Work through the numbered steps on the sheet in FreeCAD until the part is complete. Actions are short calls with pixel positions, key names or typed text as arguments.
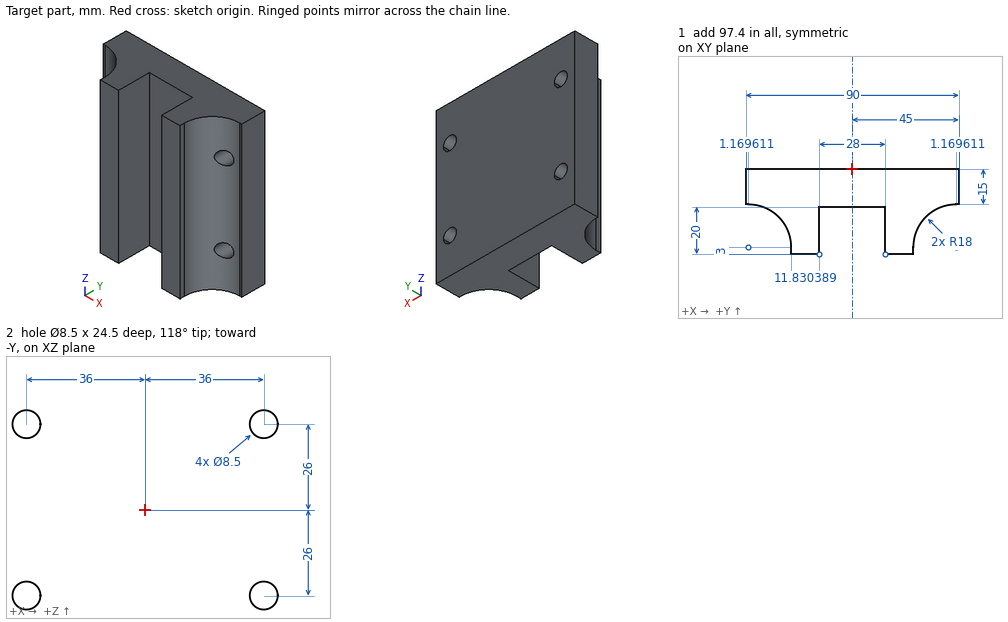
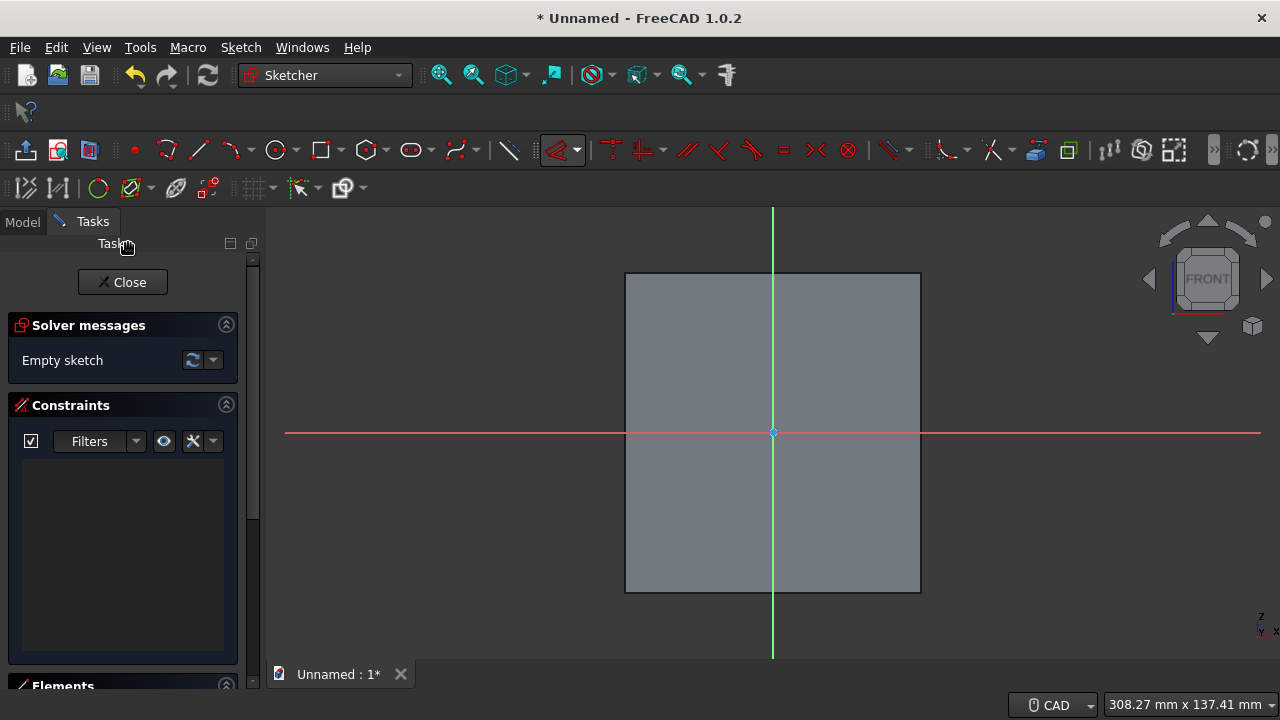
scroll(912, 433, up, 2)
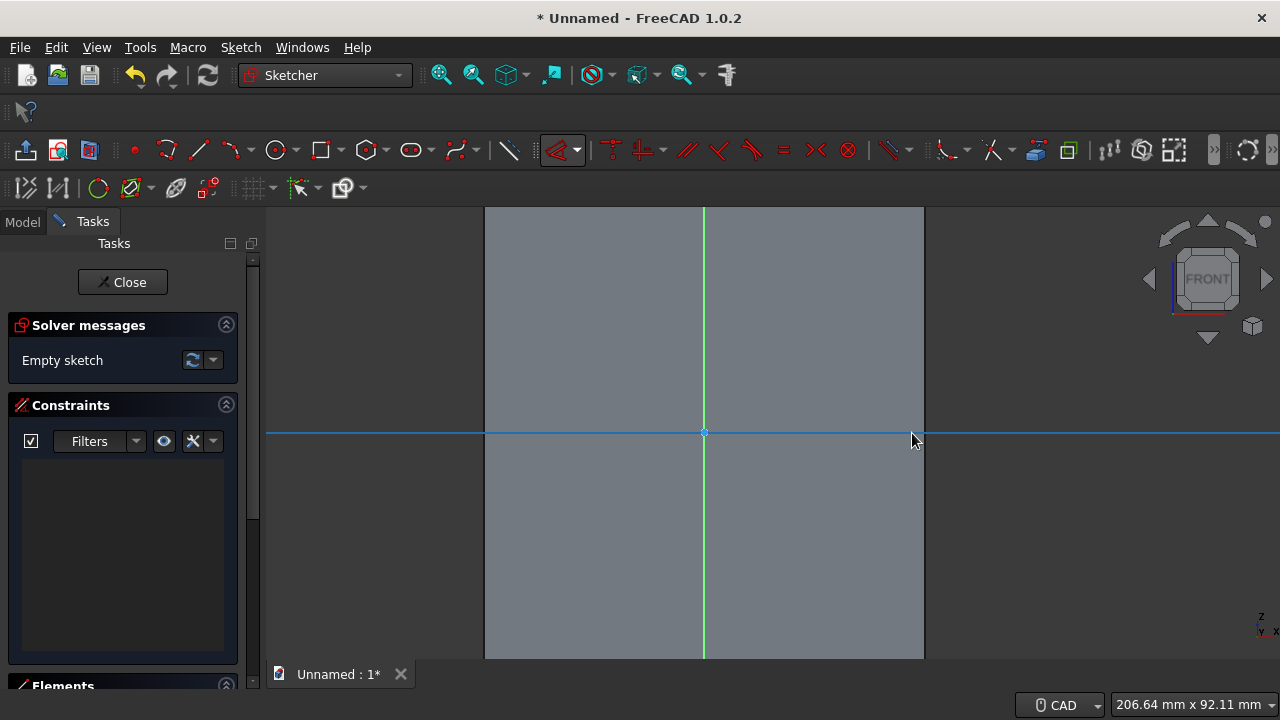
click(276, 150)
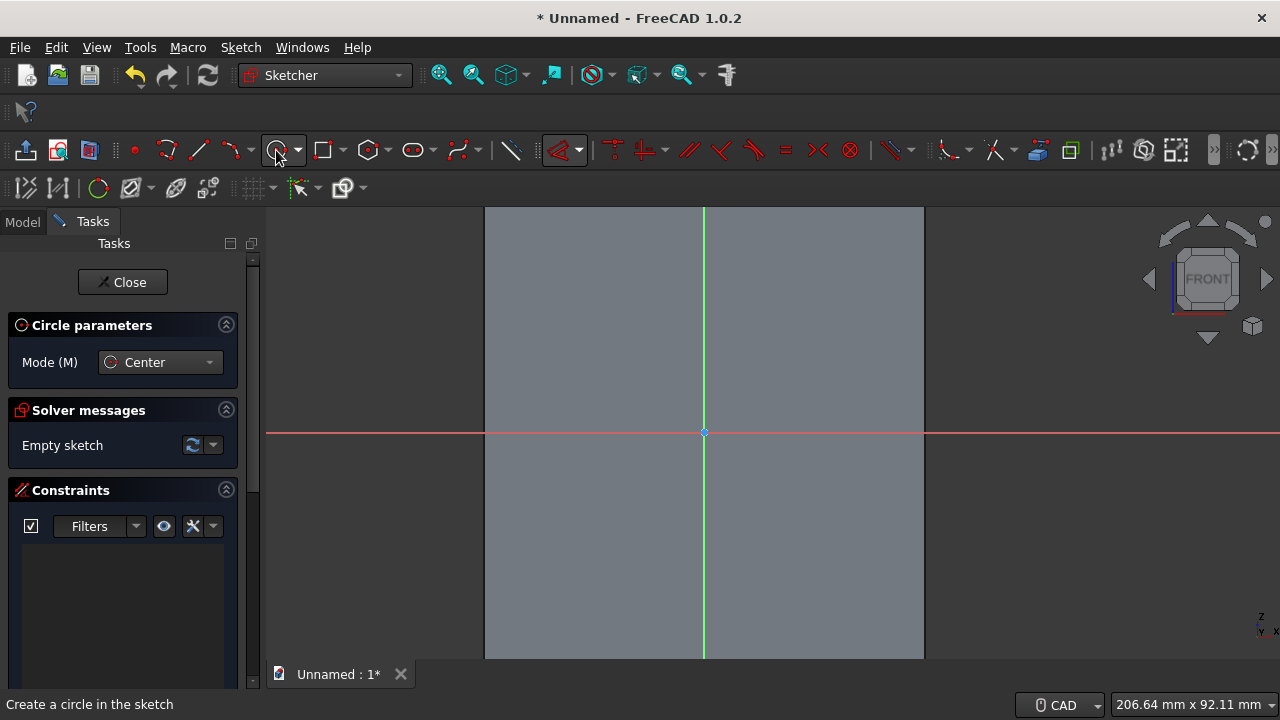
click(881, 305)
click(896, 290)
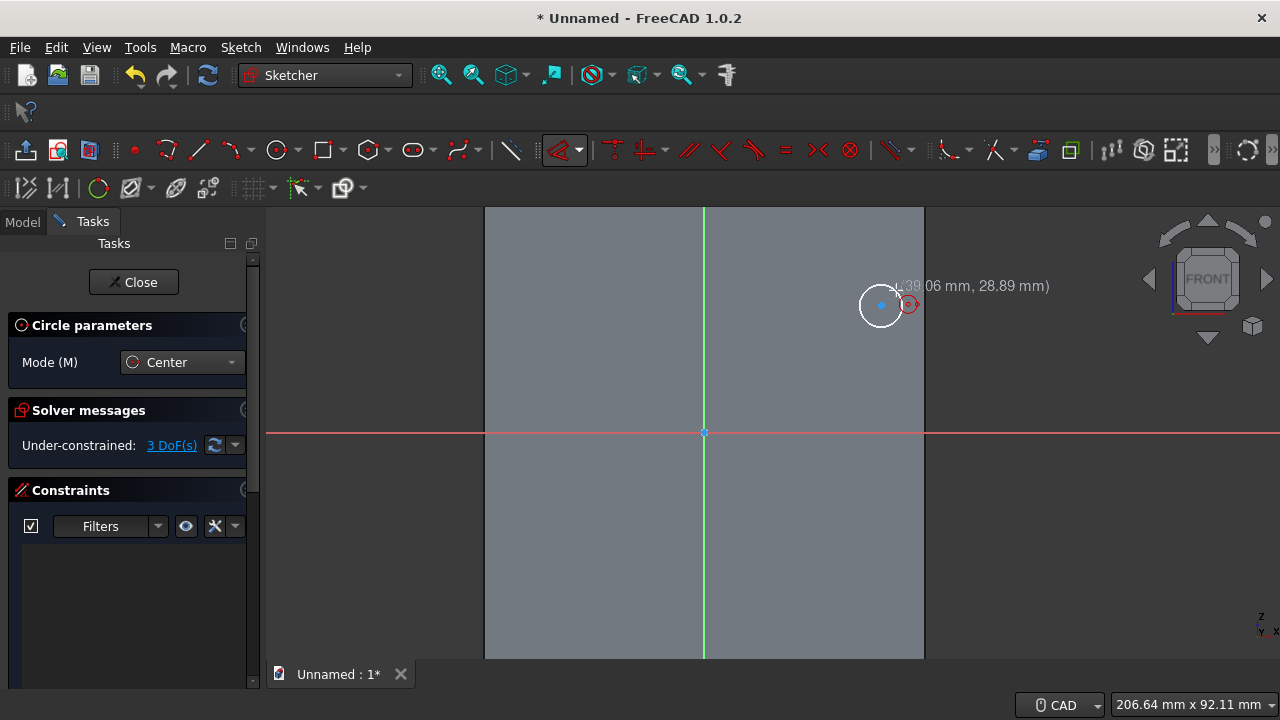
click(528, 305)
click(542, 290)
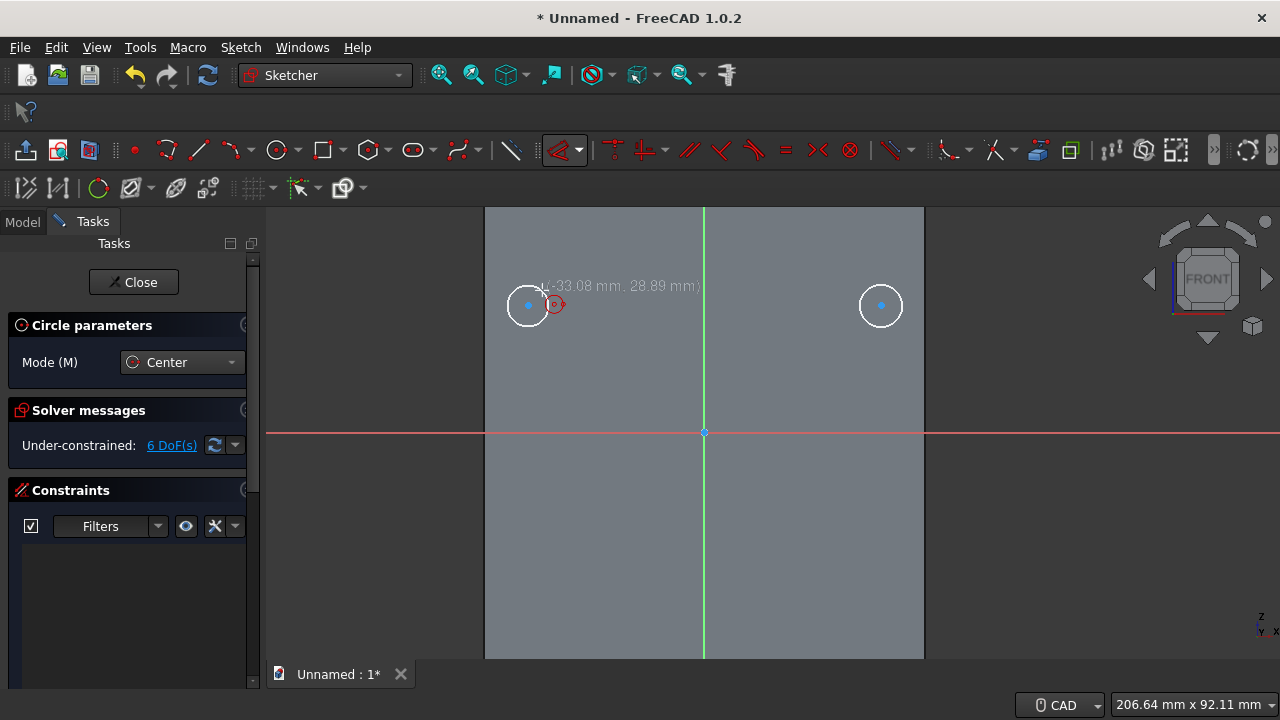
click(881, 560)
click(896, 546)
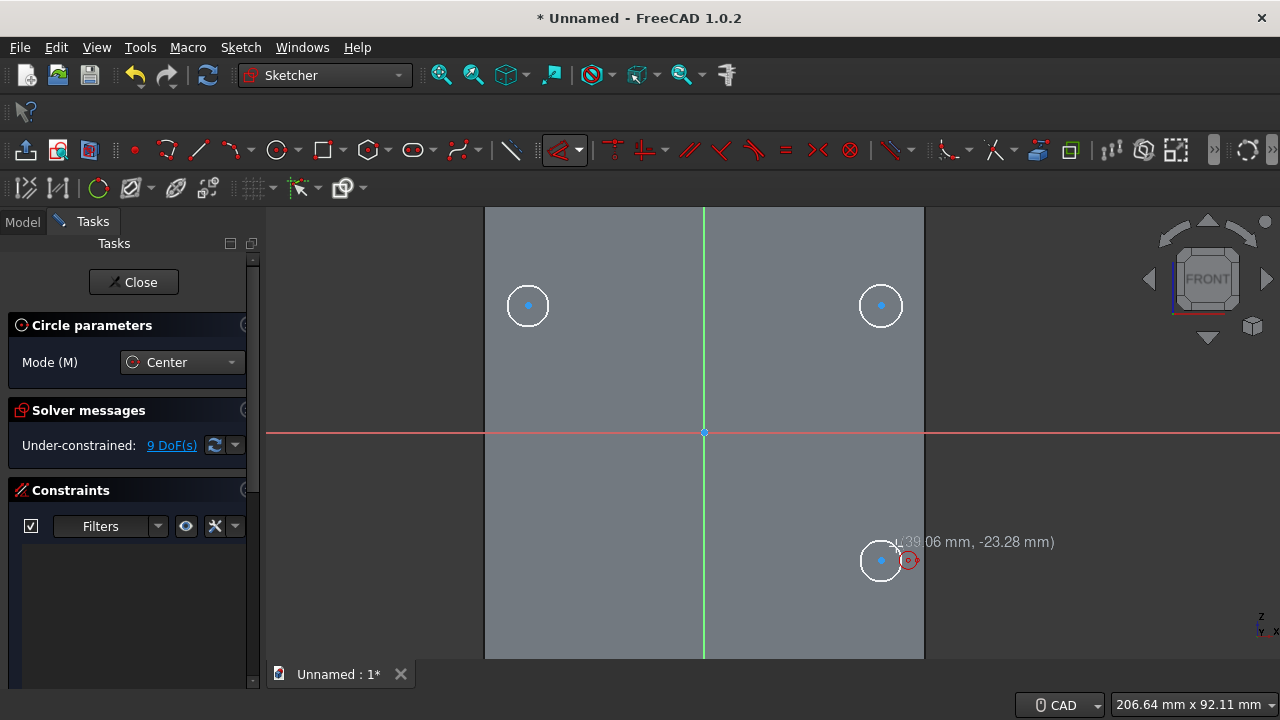
click(528, 560)
click(542, 546)
key(Escape)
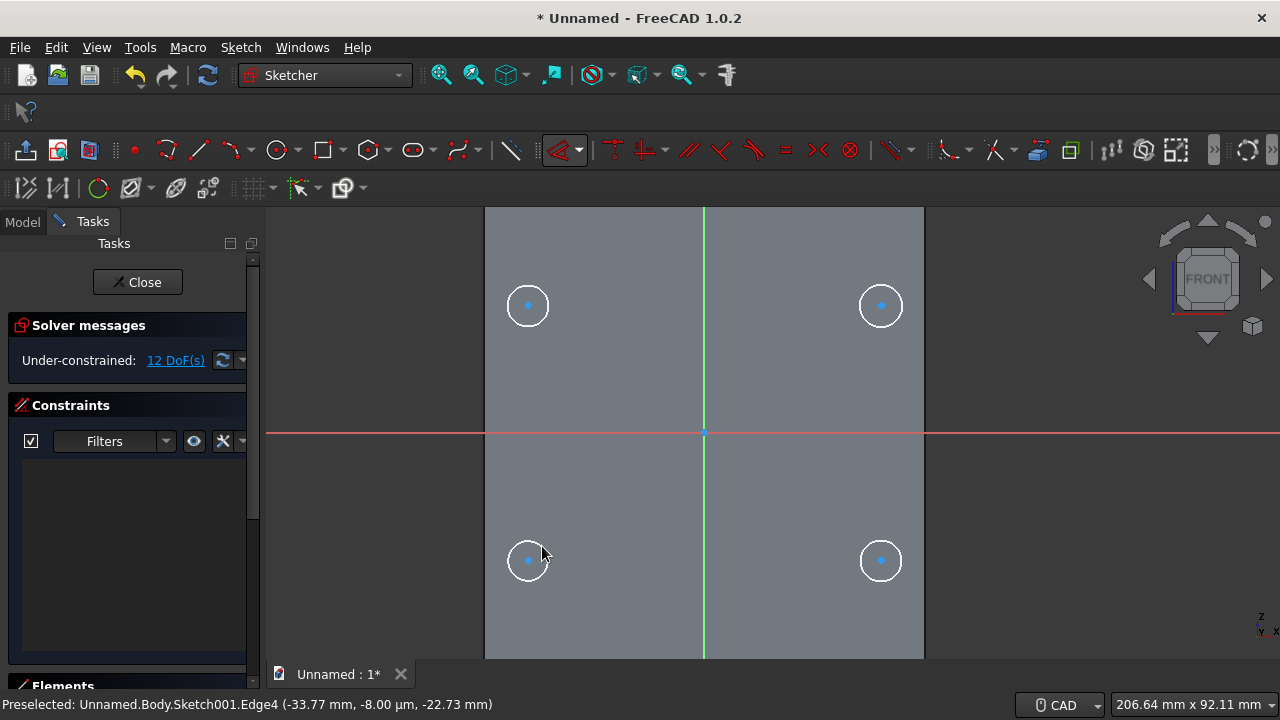
click(896, 291)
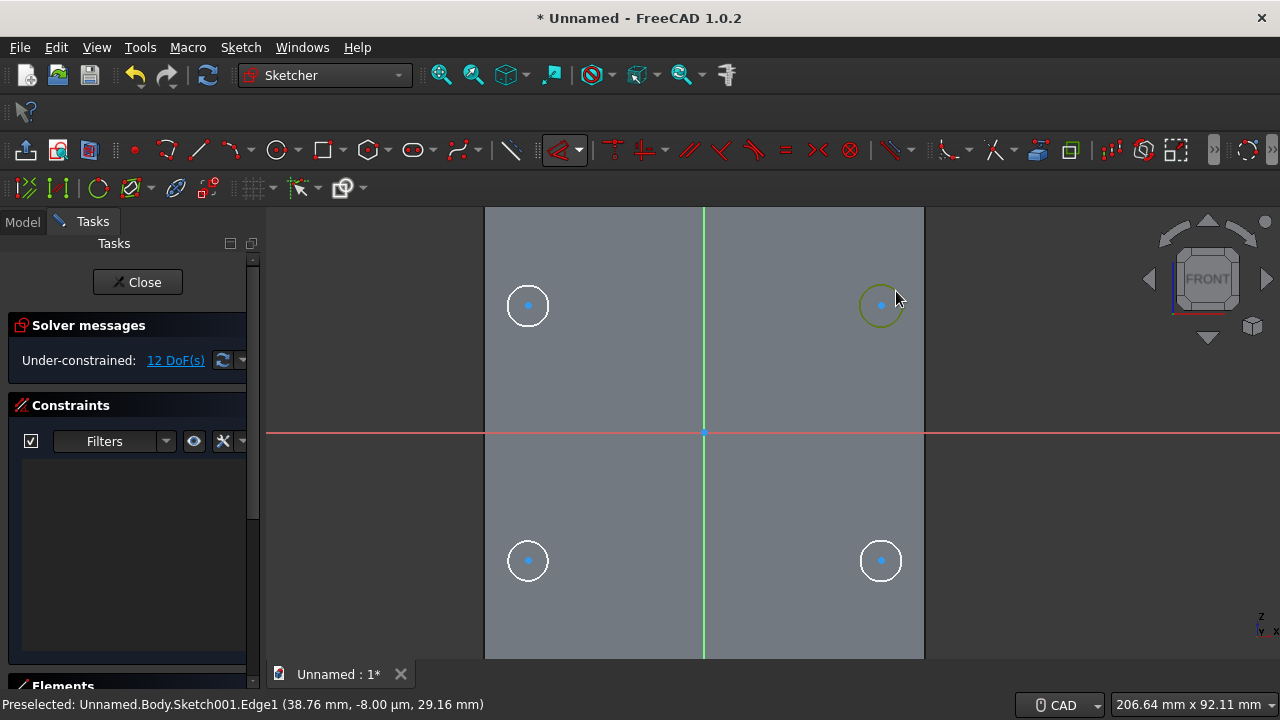
click(542, 291)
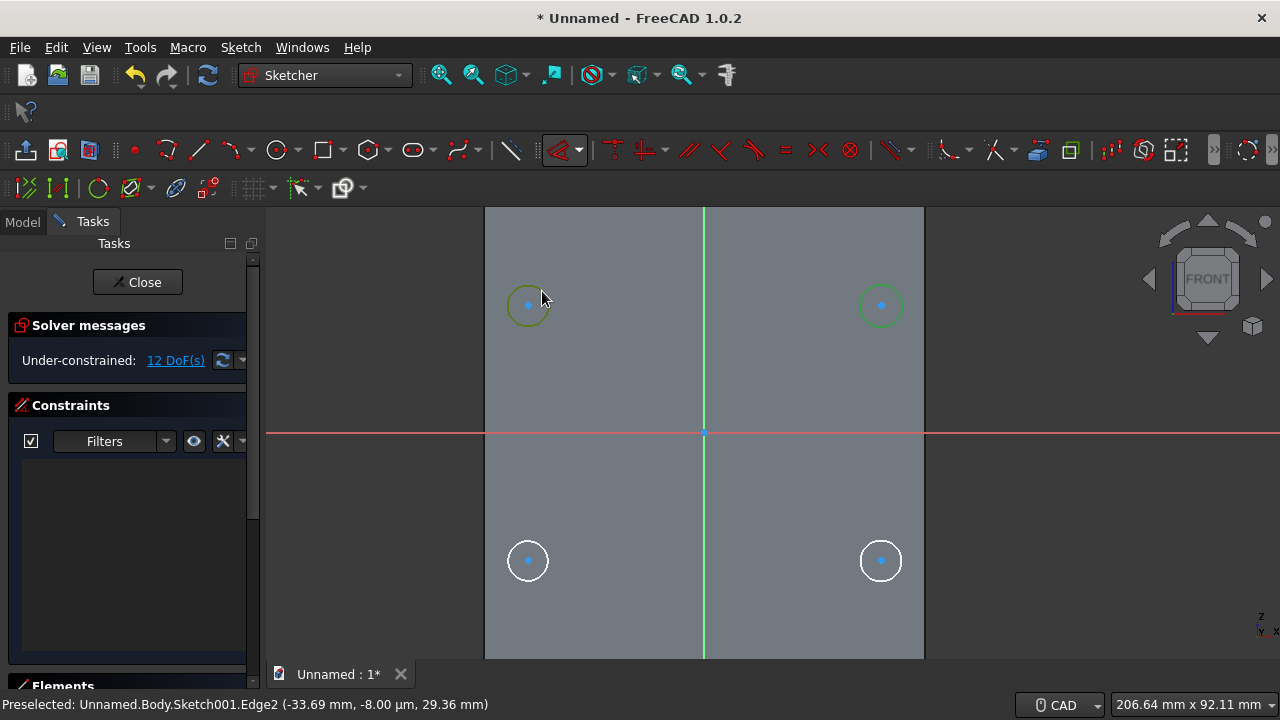
click(895, 546)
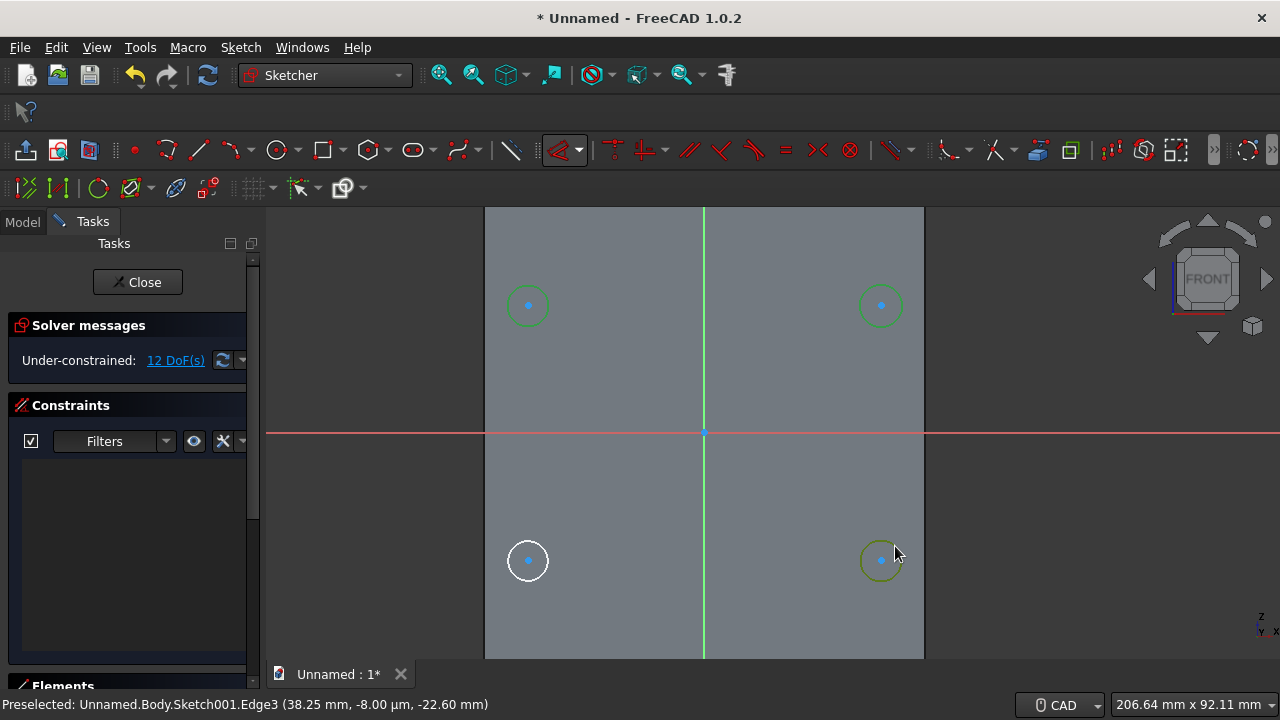
click(542, 547)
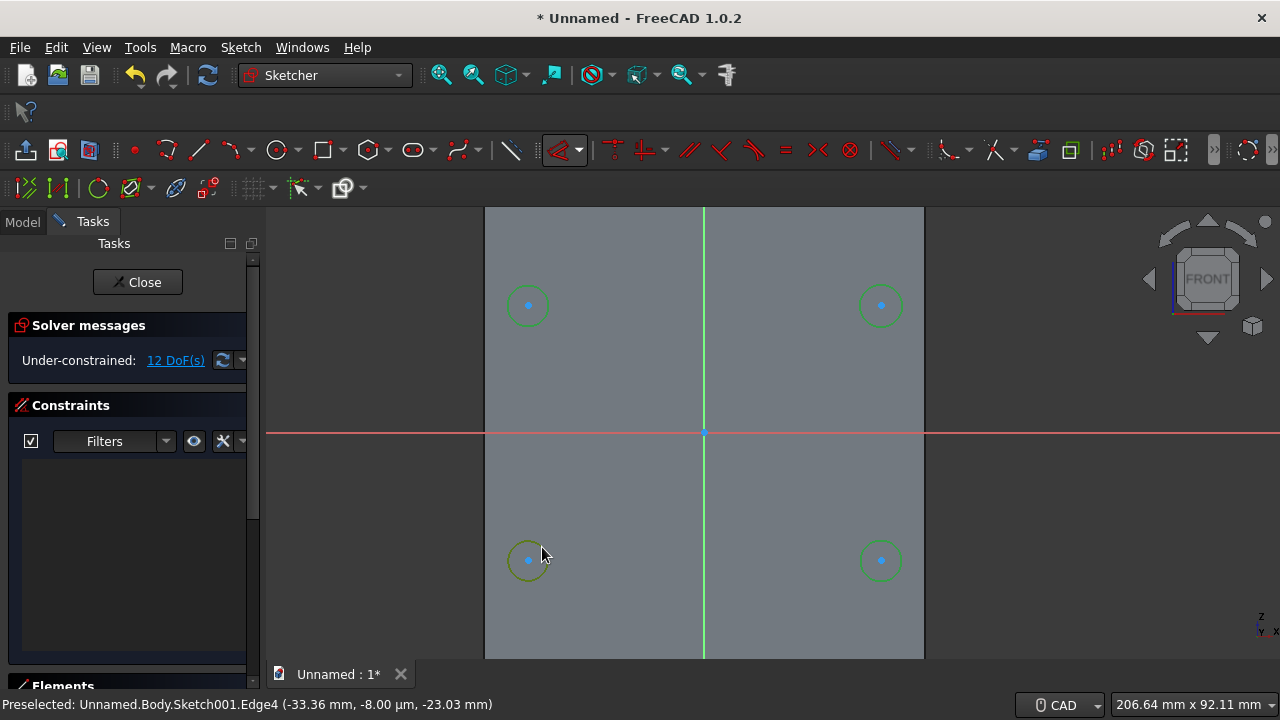
click(786, 150)